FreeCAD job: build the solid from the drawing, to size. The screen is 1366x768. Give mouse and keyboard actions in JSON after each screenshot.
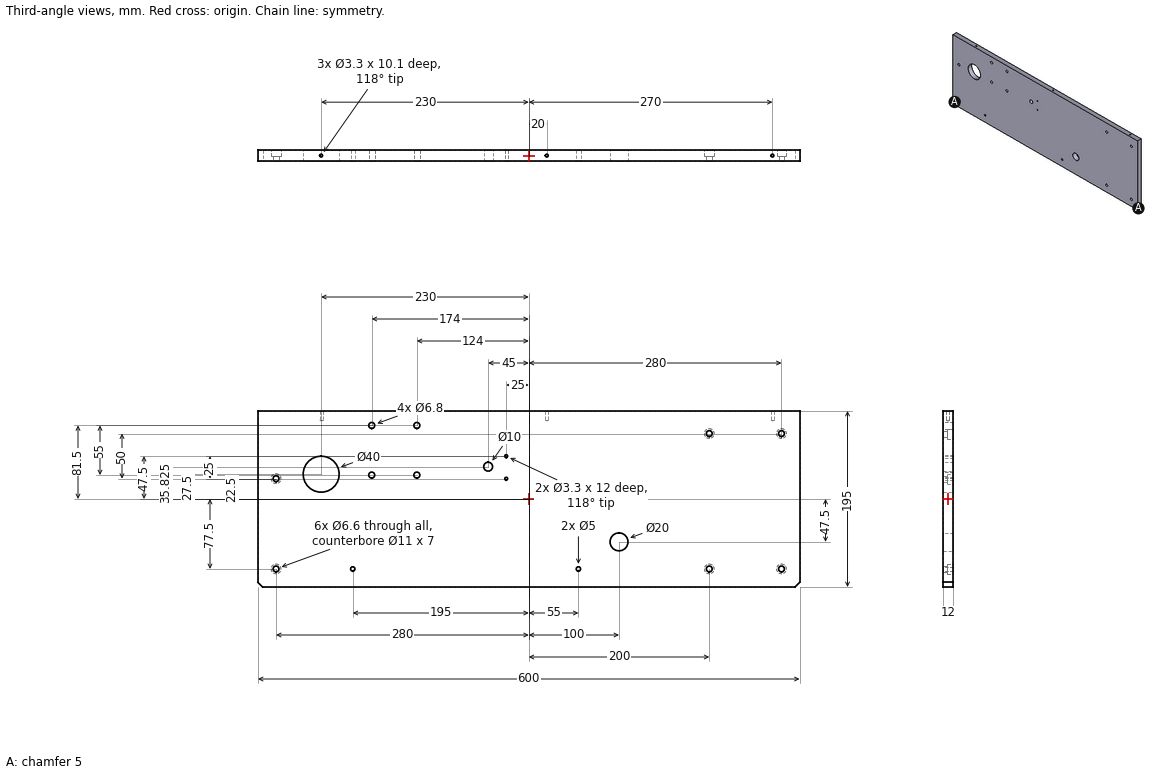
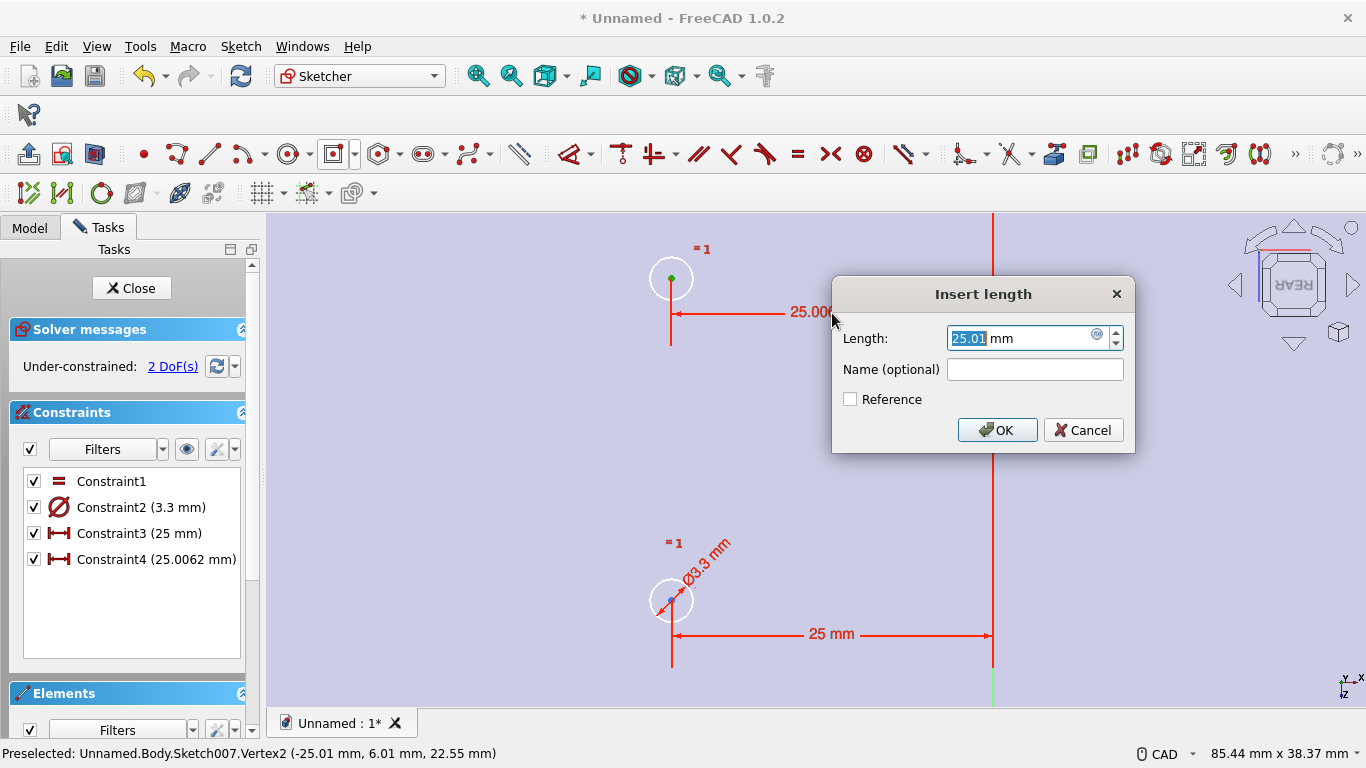
{"action": "type", "text": "25"}
{"action": "key", "text": "Return"}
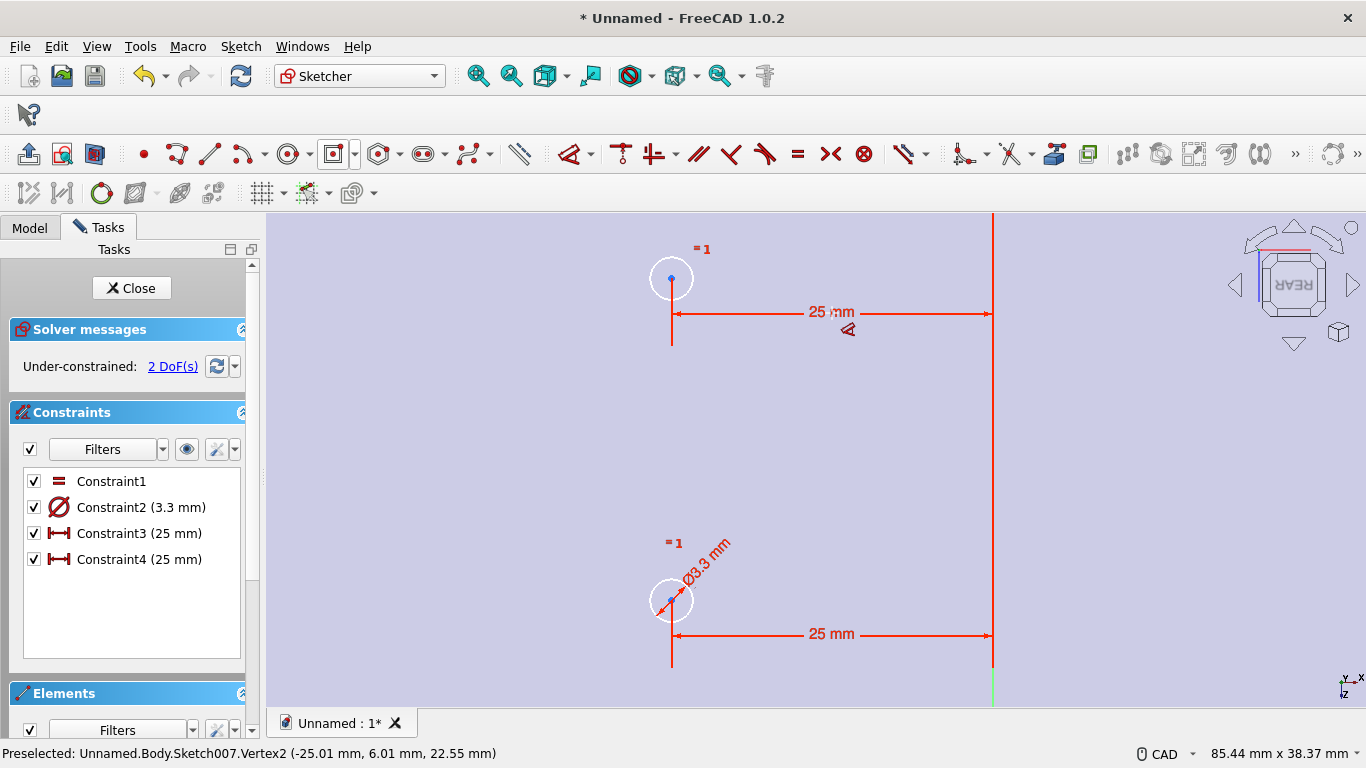
{"action": "left_click", "coordinate": [672, 601]}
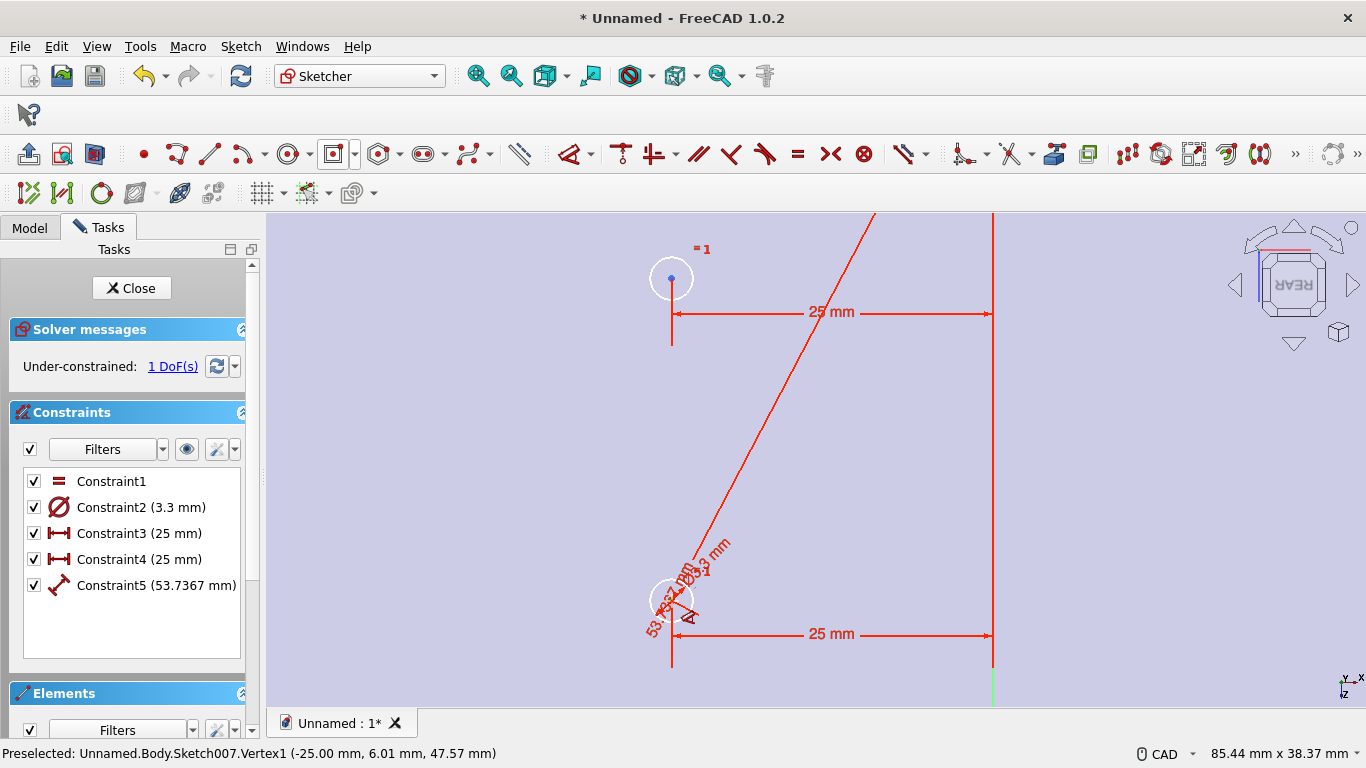
{"action": "left_click", "coordinate": [672, 279]}
{"action": "left_click", "coordinate": [638, 440]}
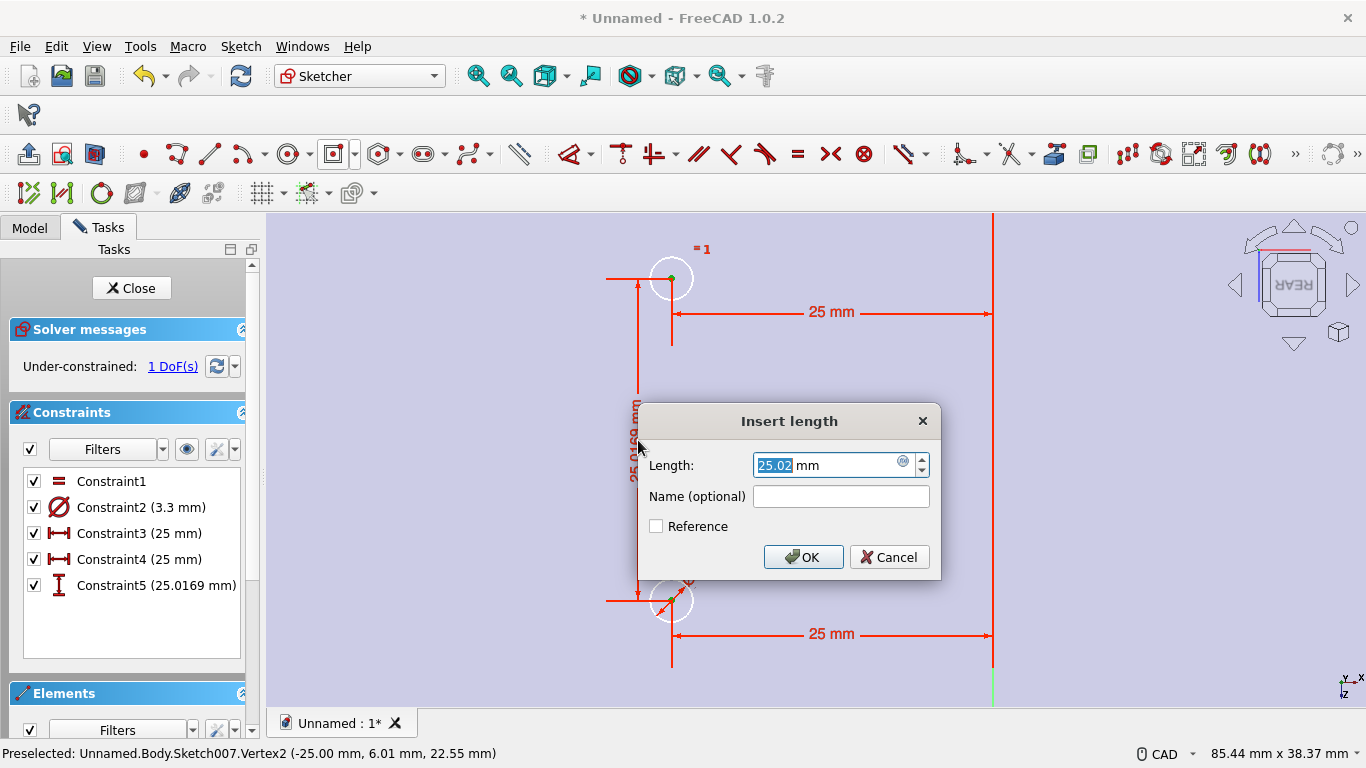
{"action": "type", "text": "25"}
{"action": "key", "text": "Return"}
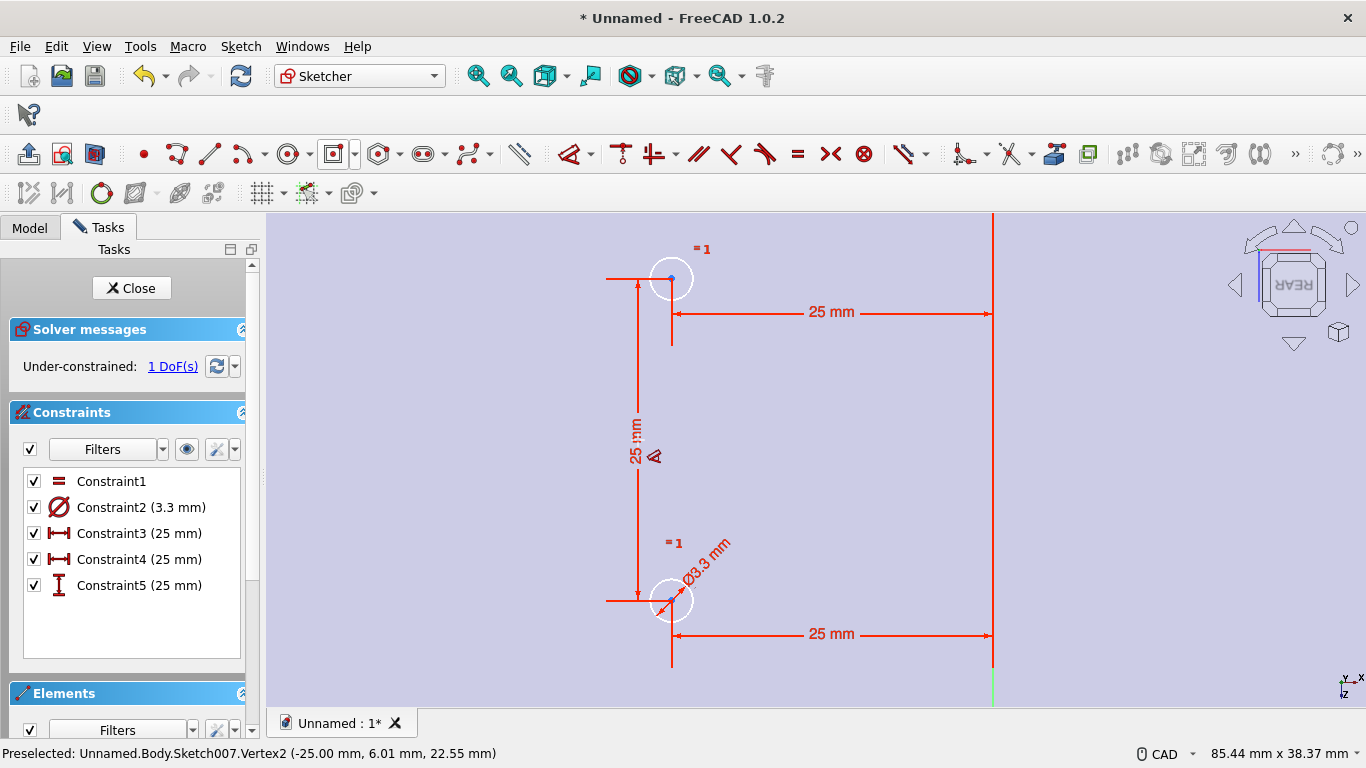
{"action": "left_click", "coordinate": [672, 601]}
{"action": "left_click", "coordinate": [1027, 421]}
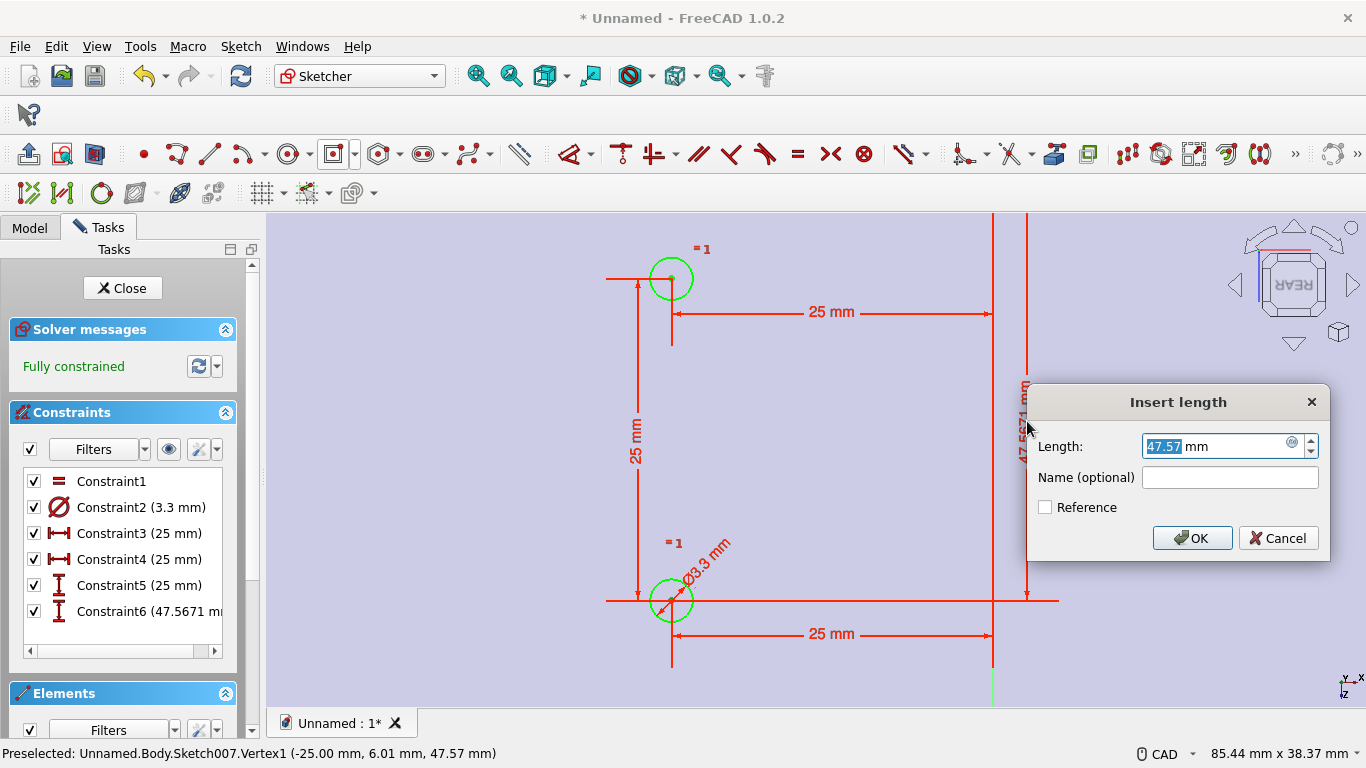
{"action": "type", "text": "47.5"}
{"action": "key", "text": "Return"}
{"action": "key", "text": "Escape"}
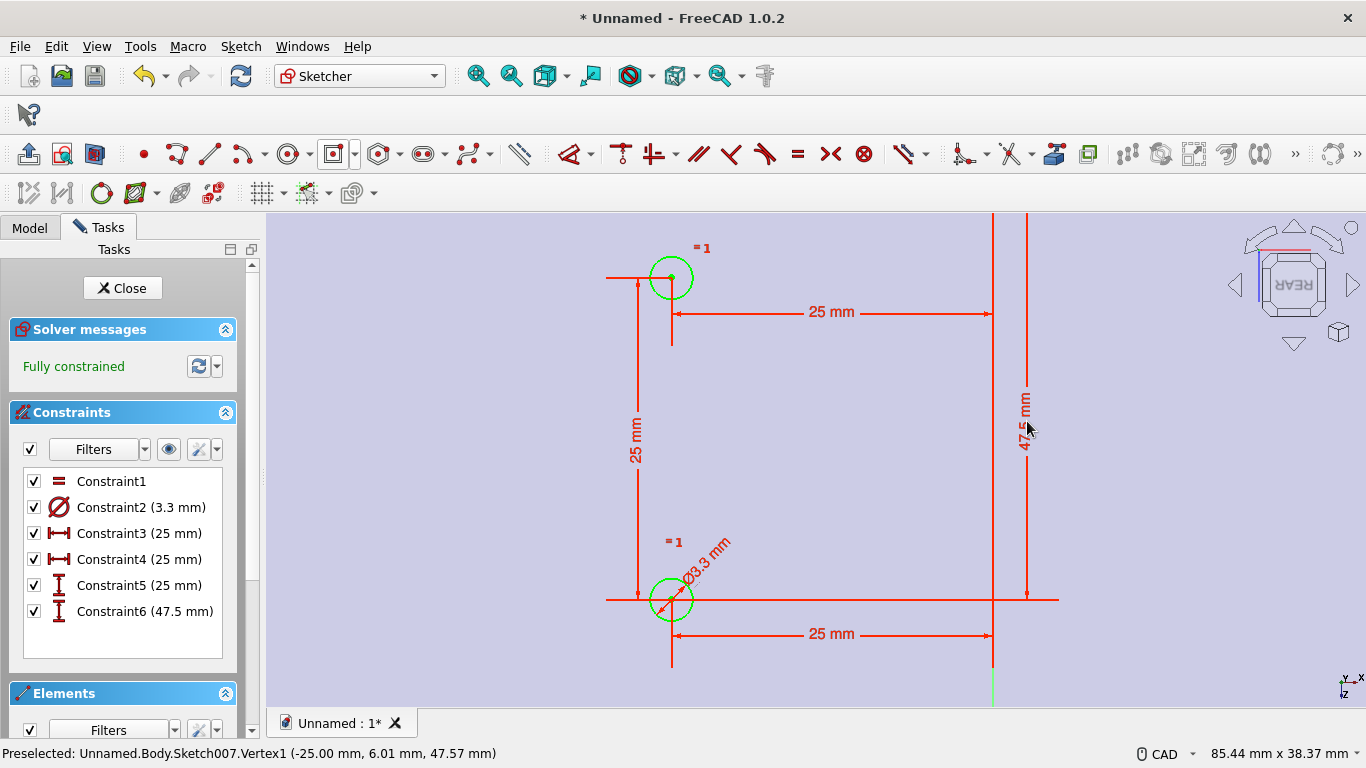
{"action": "left_click", "coordinate": [123, 288]}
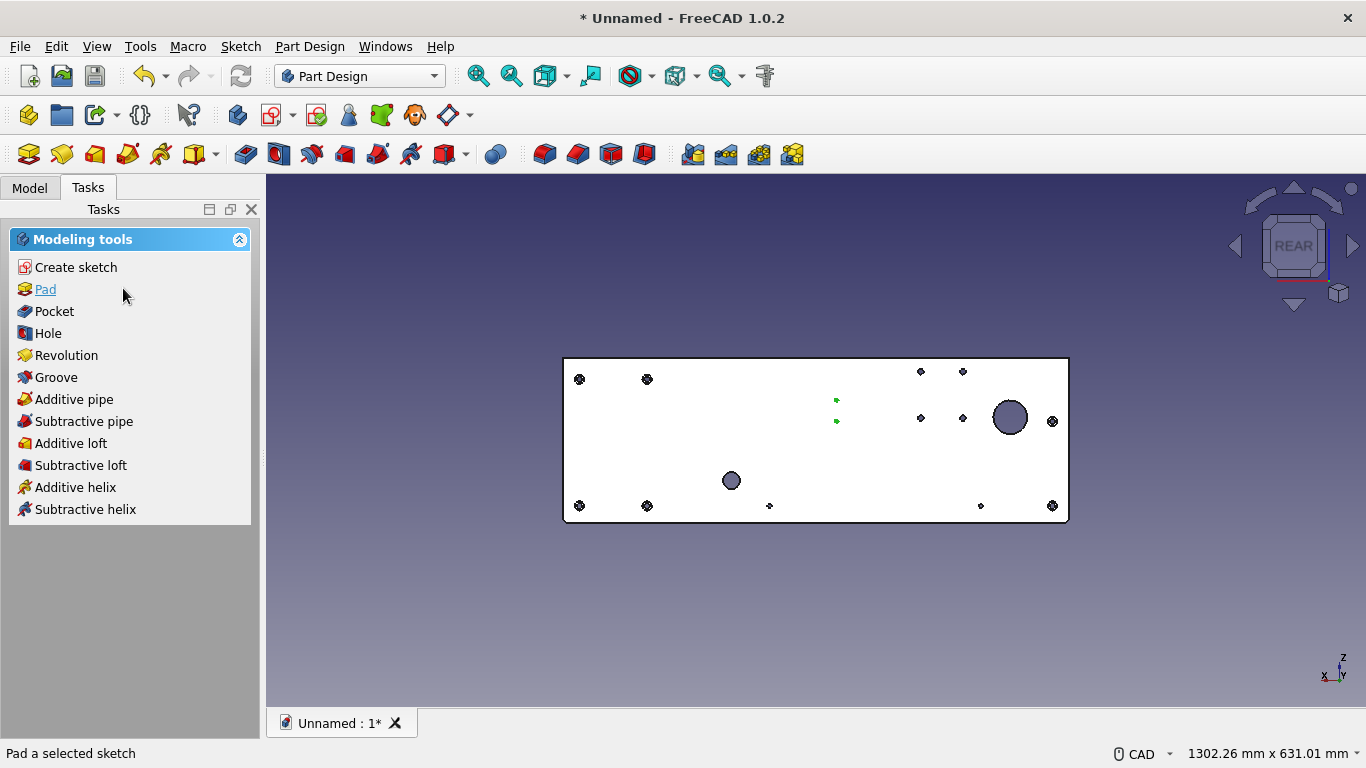
{"action": "left_click", "coordinate": [279, 154]}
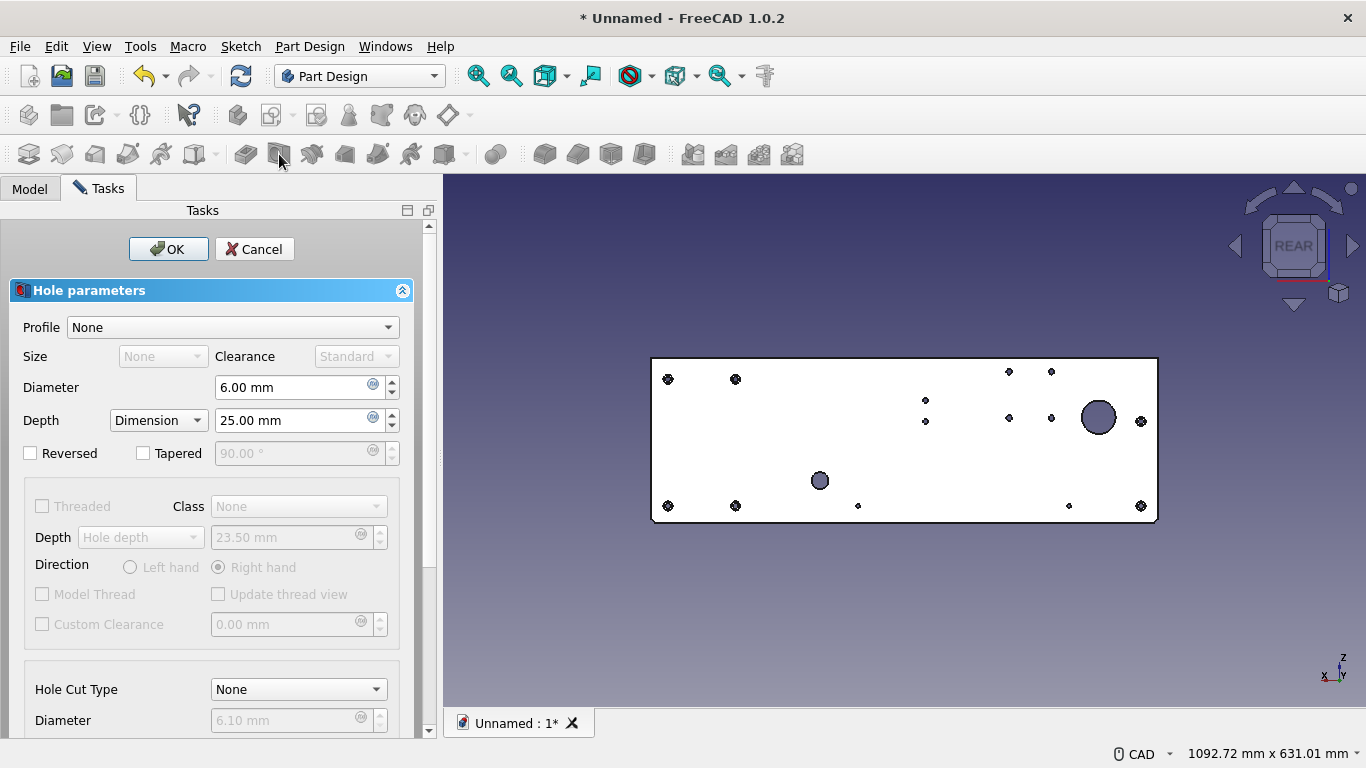
{"action": "triple_click", "coordinate": [300, 388]}